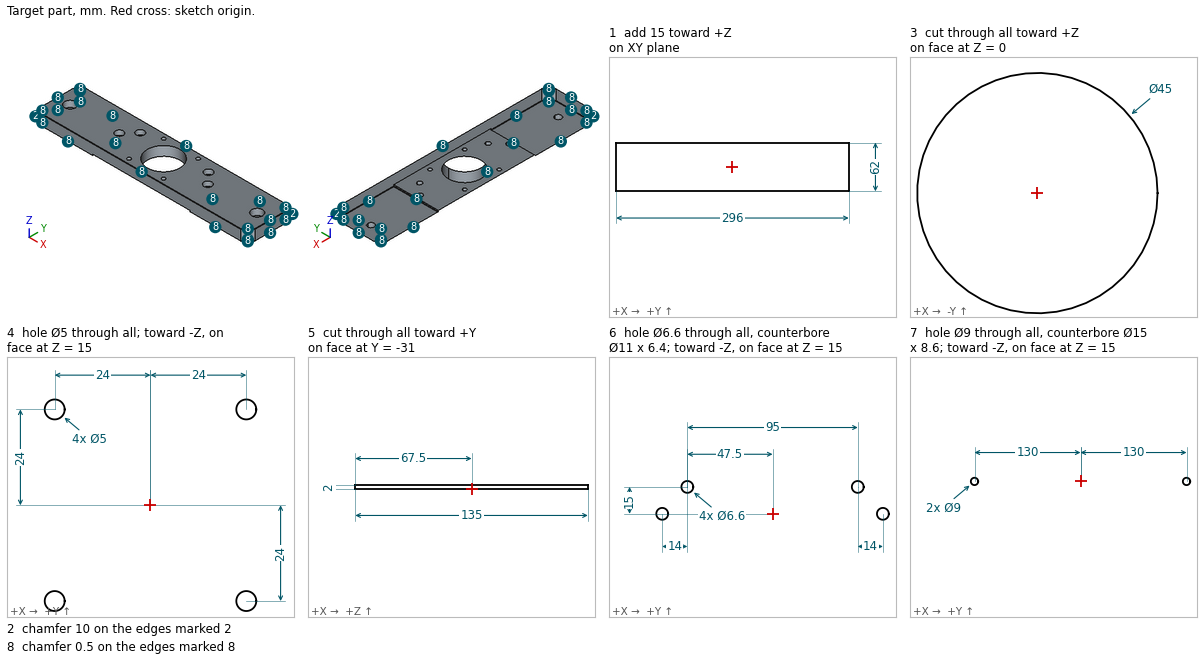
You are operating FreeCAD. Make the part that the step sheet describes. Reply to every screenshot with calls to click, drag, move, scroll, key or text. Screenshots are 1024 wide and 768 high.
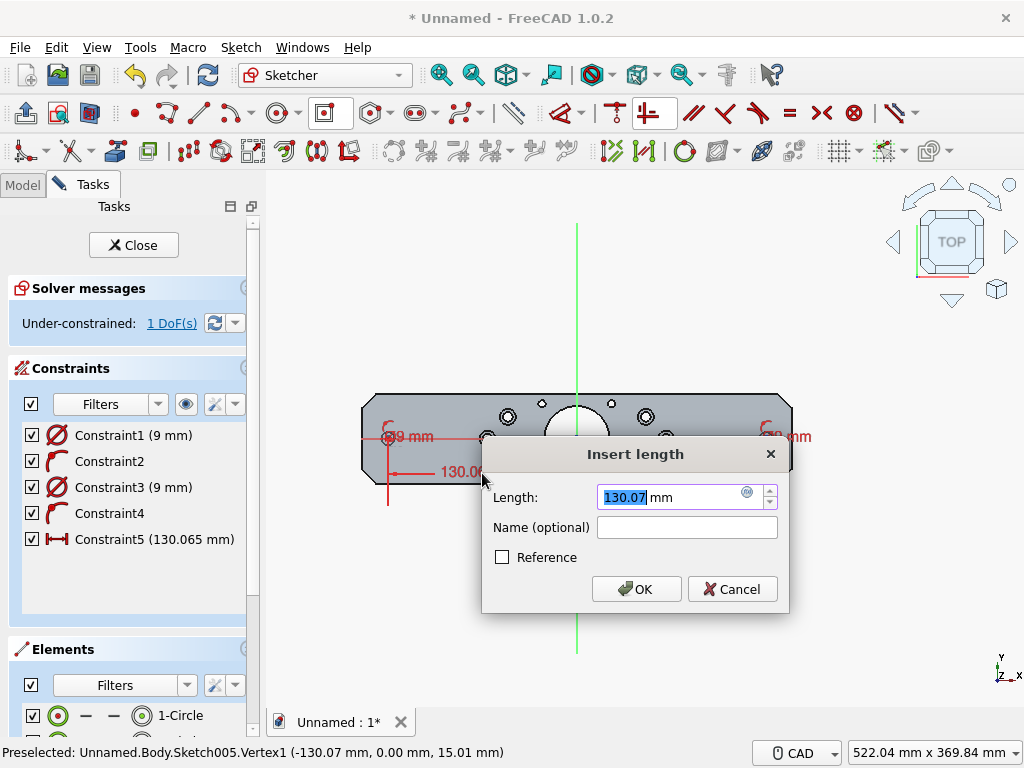
text(130)
key(Return)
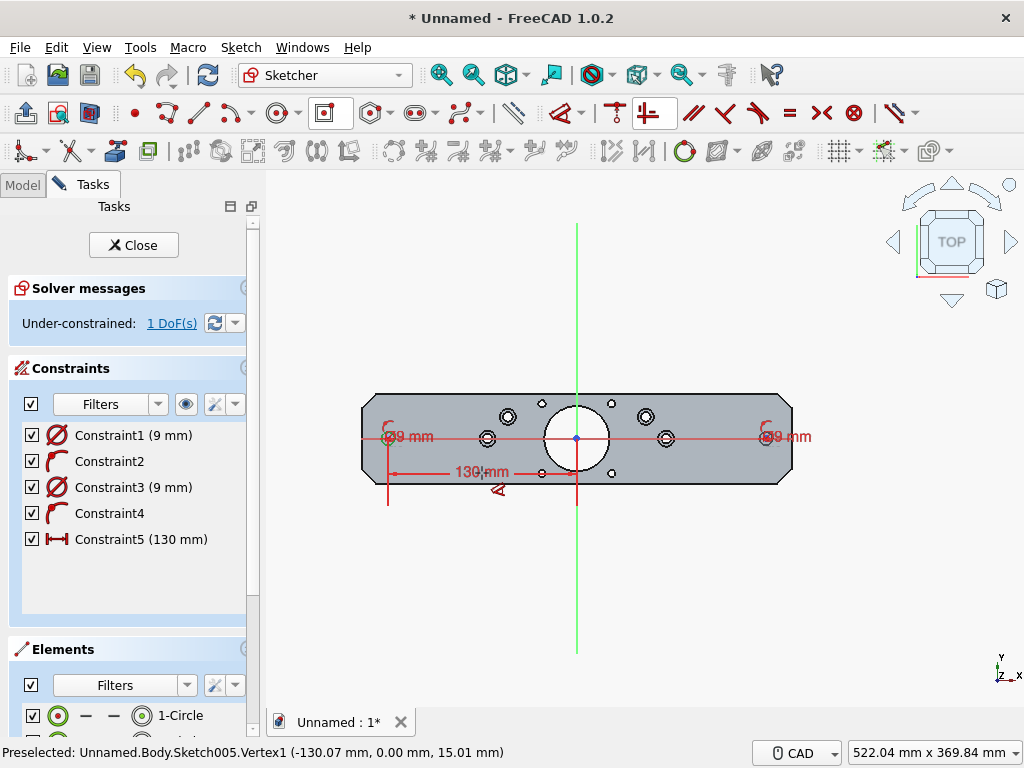
click(766, 439)
click(671, 473)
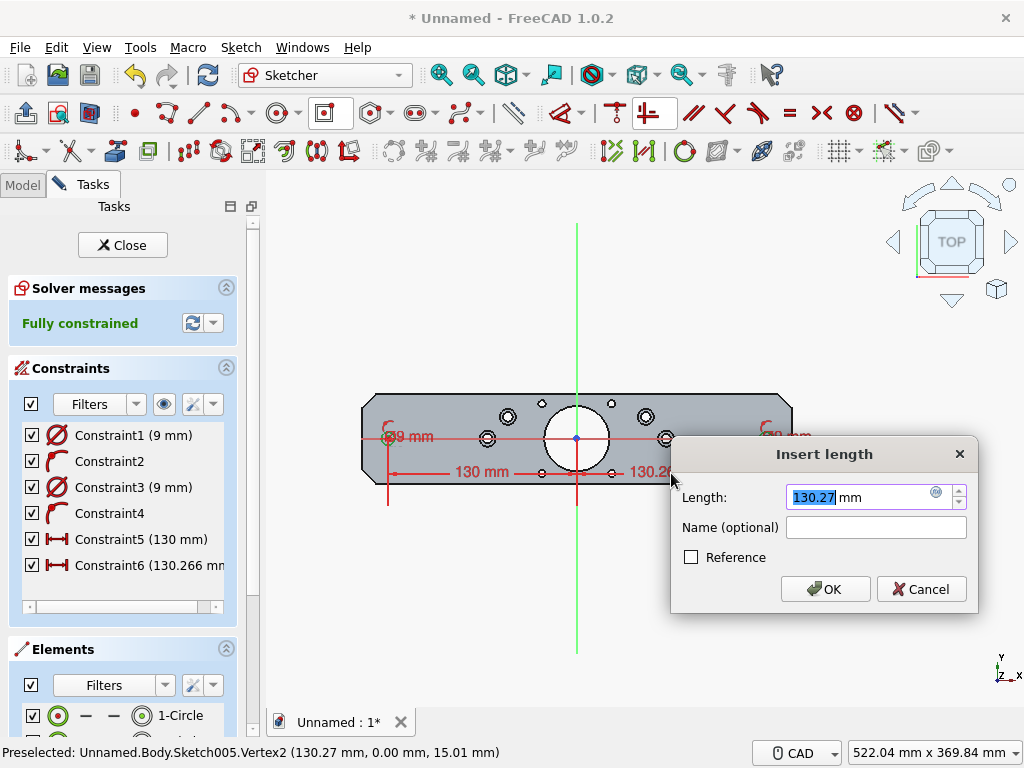
text(130)
key(Return)
key(Escape)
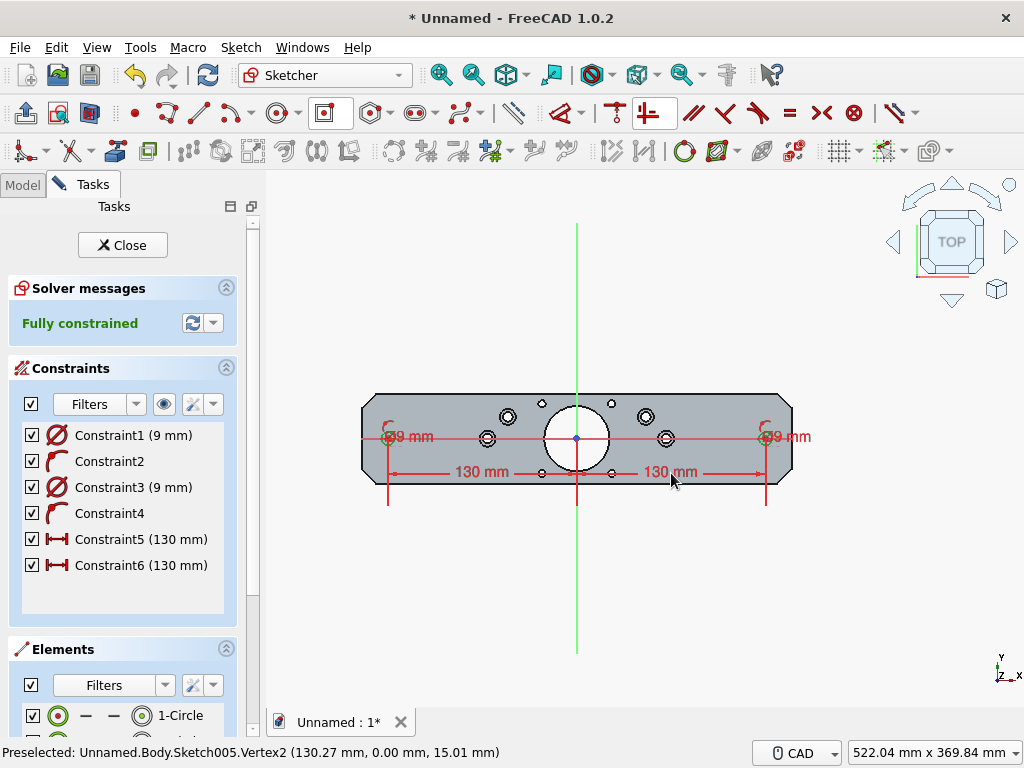
click(123, 245)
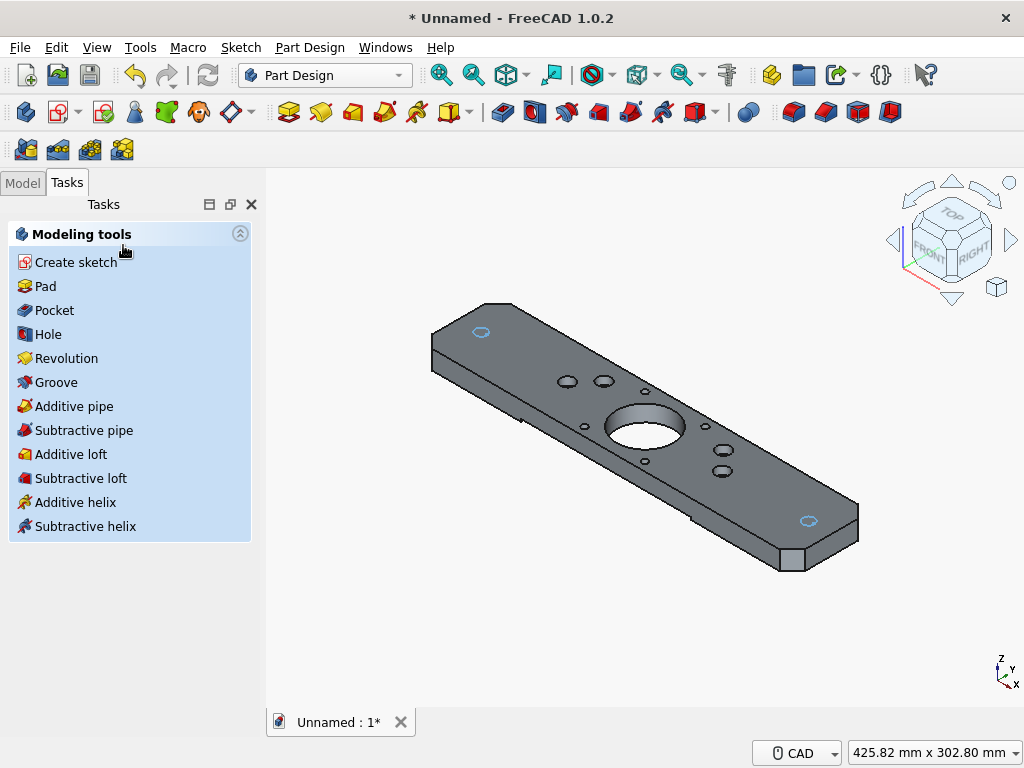
click(536, 112)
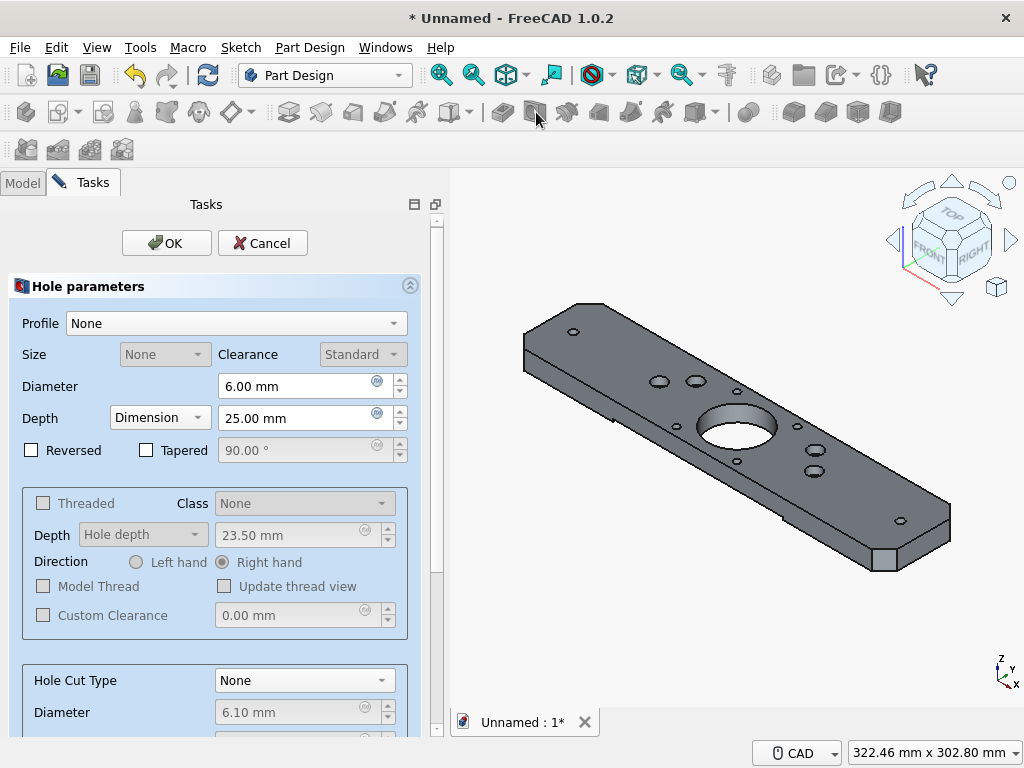
triple_click(305, 386)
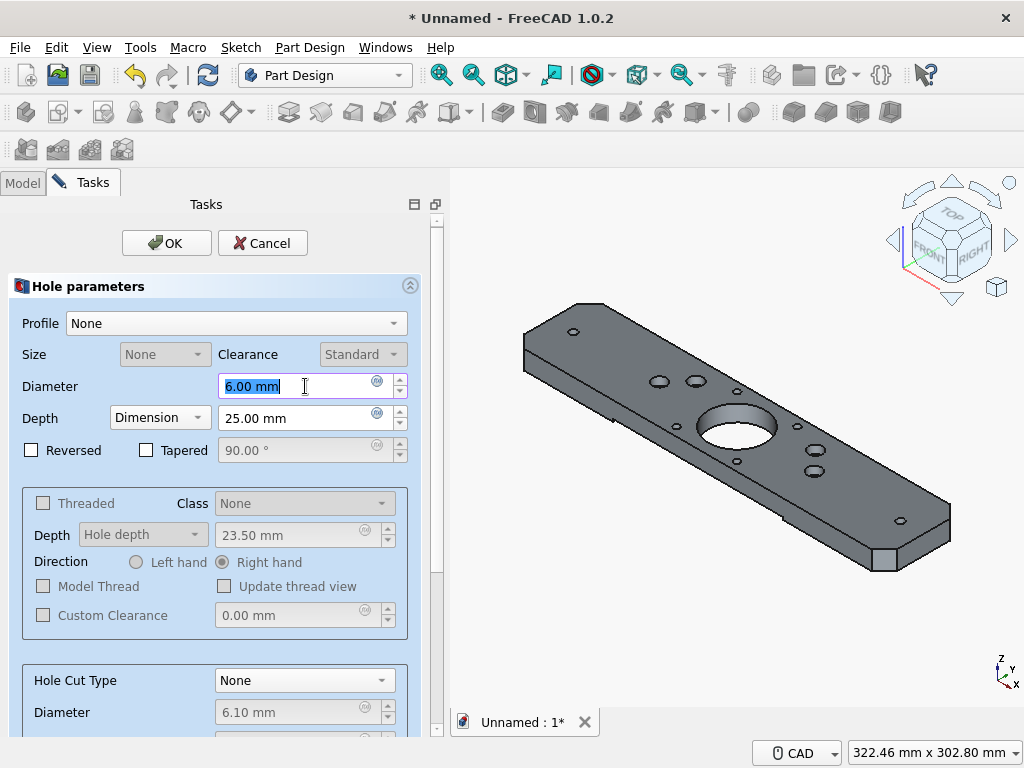
text(9)
key(Tab)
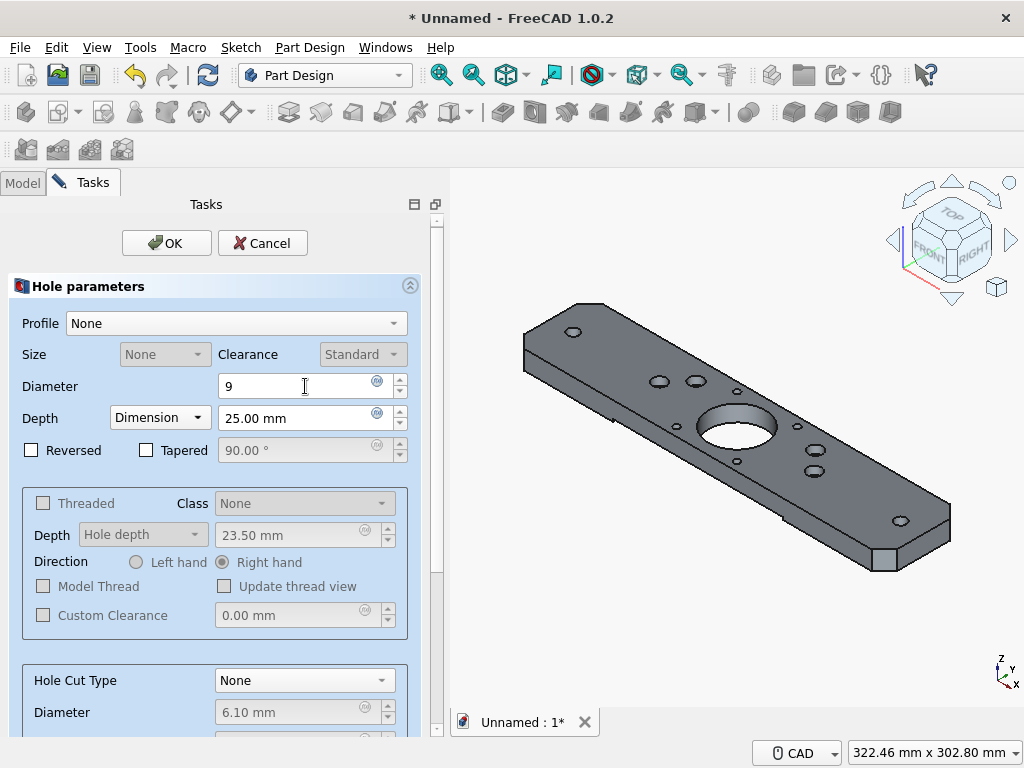
click(161, 418)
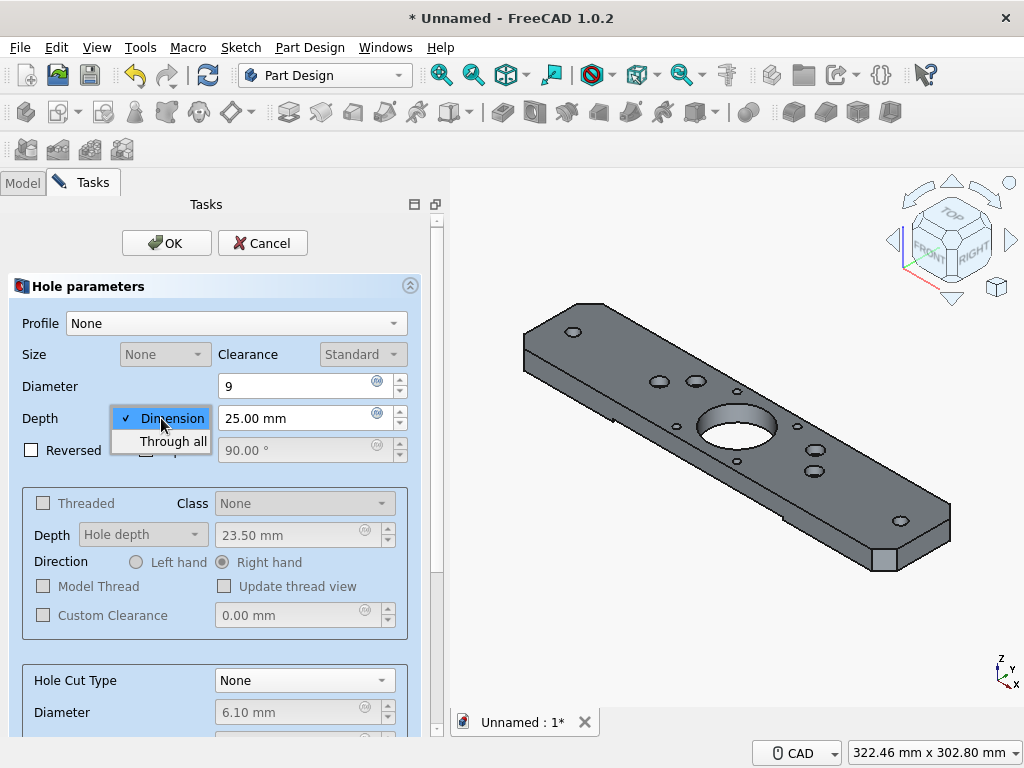
click(160, 442)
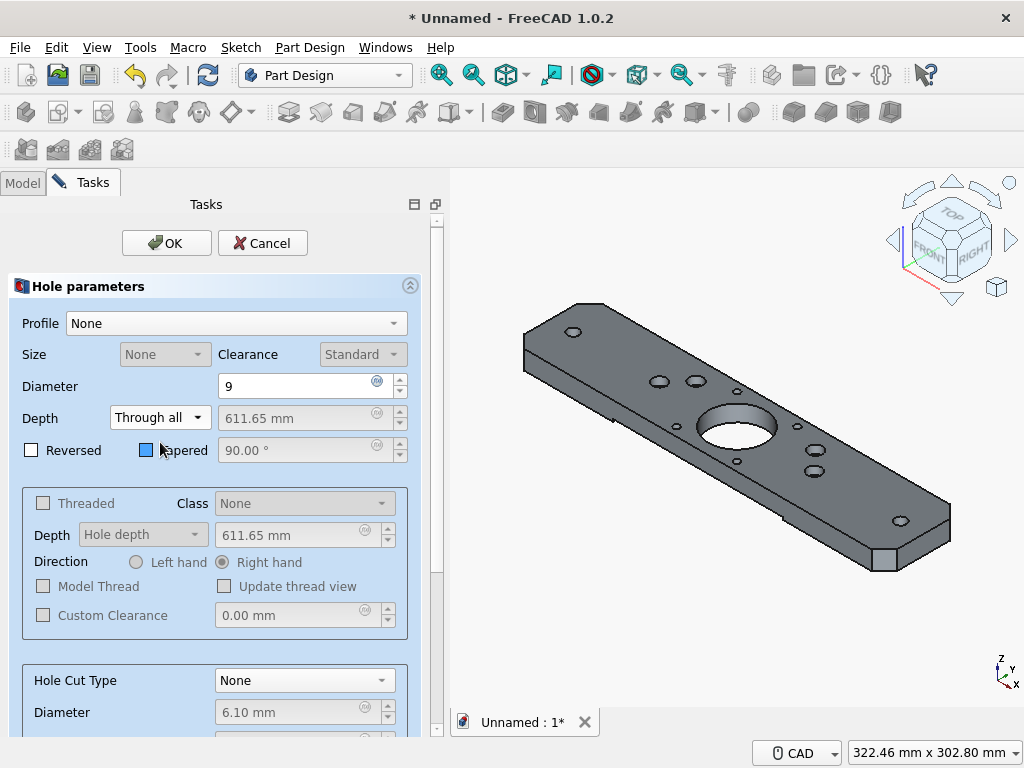
click(306, 680)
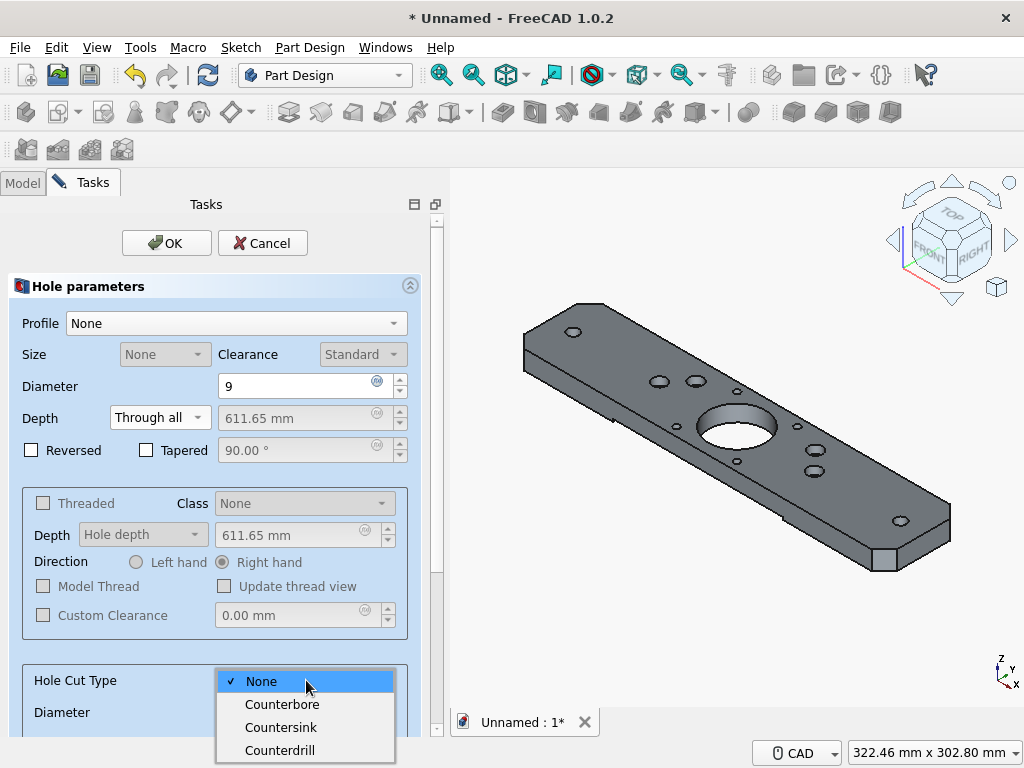
click(304, 704)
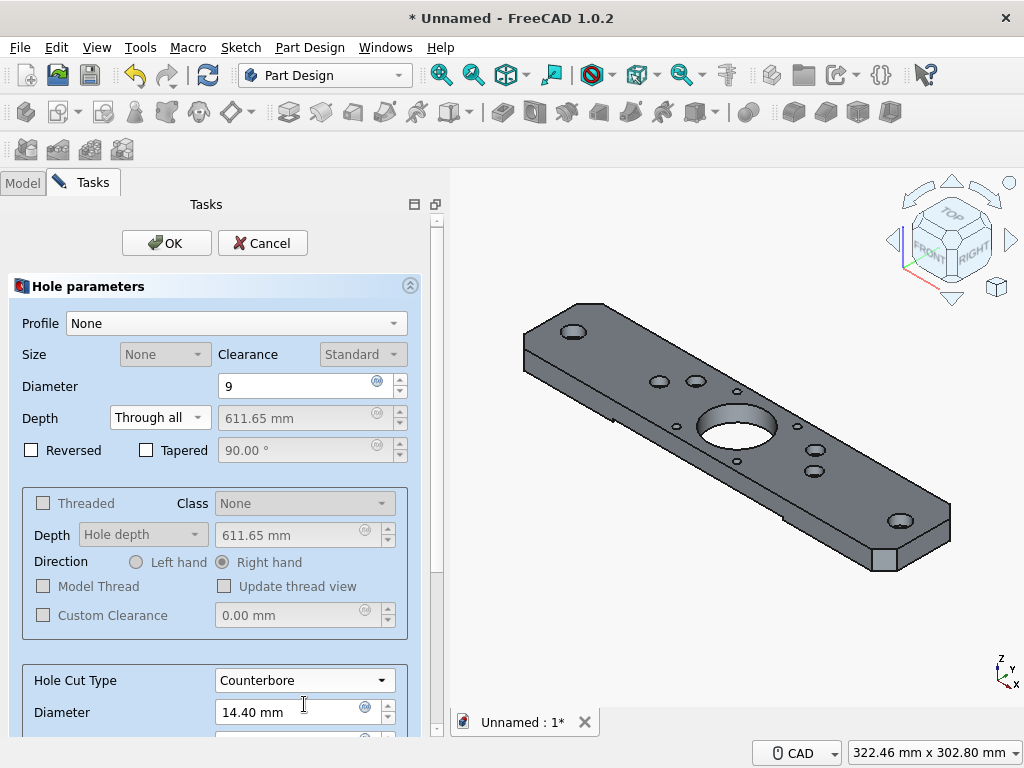
triple_click(298, 712)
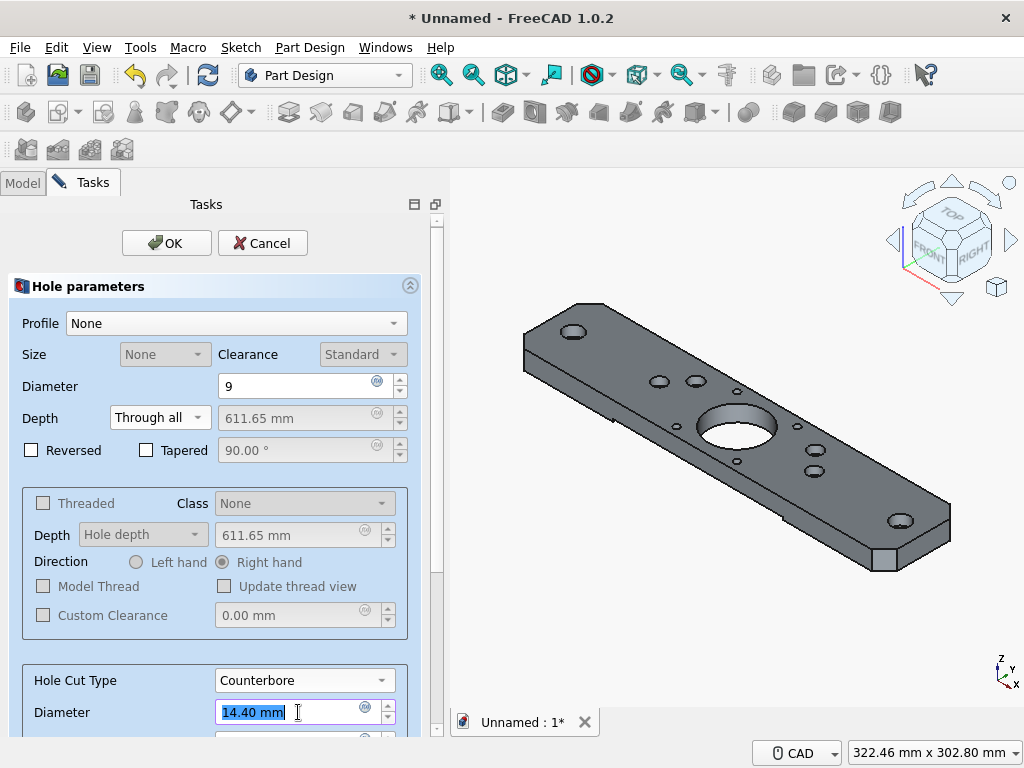
text(15)
key(Tab)